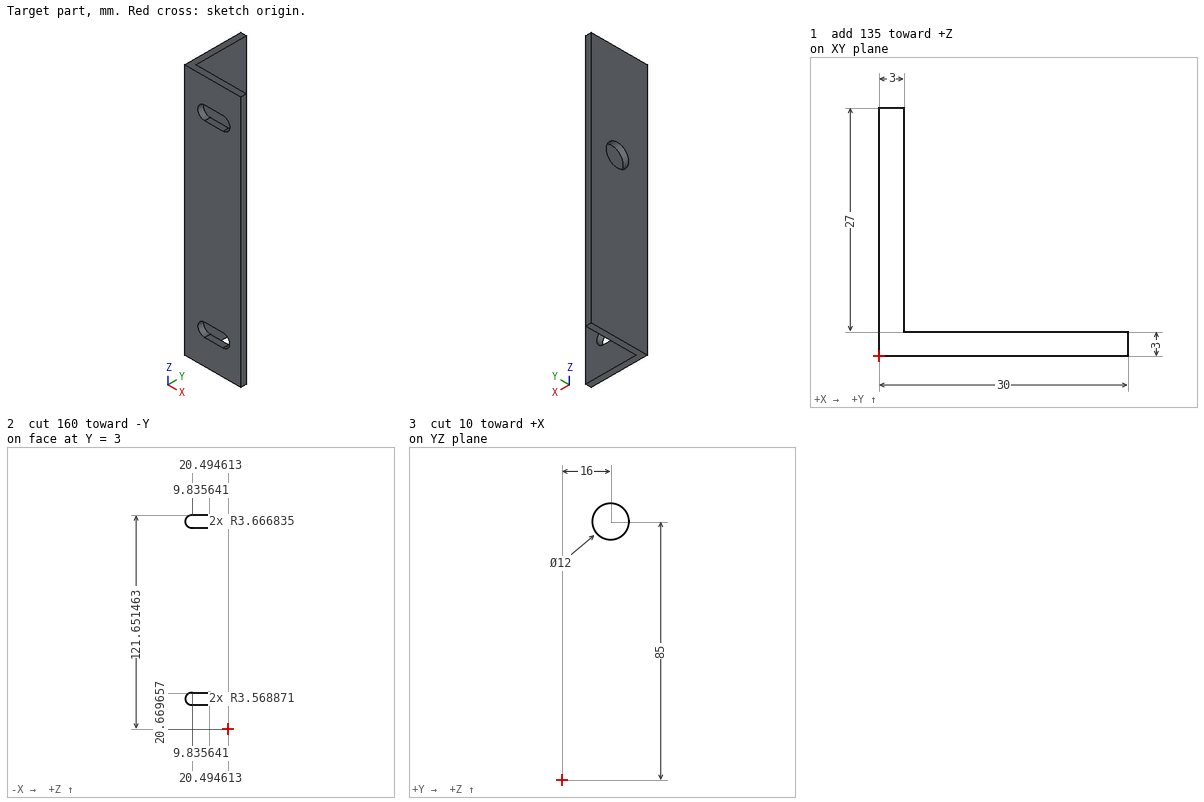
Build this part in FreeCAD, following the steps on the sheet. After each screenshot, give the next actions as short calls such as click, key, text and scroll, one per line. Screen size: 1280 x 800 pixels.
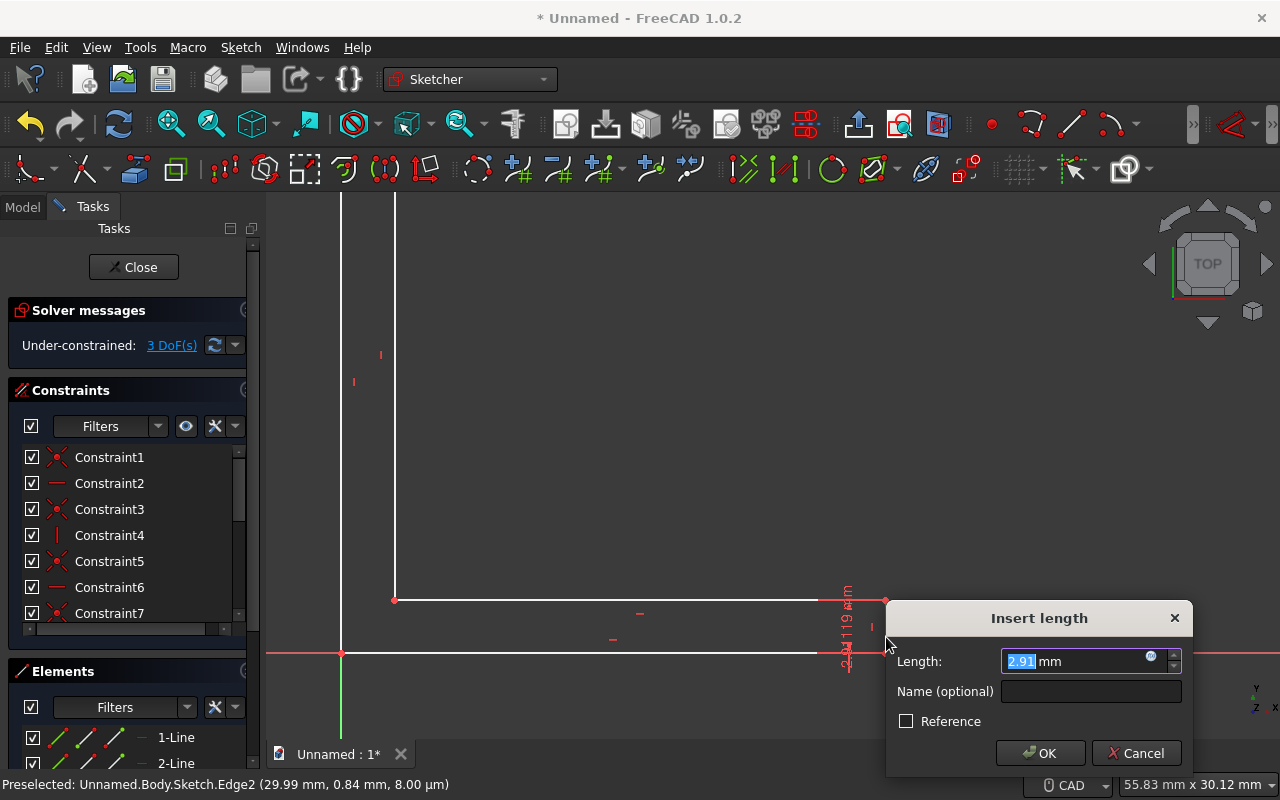
text(3)
key(Return)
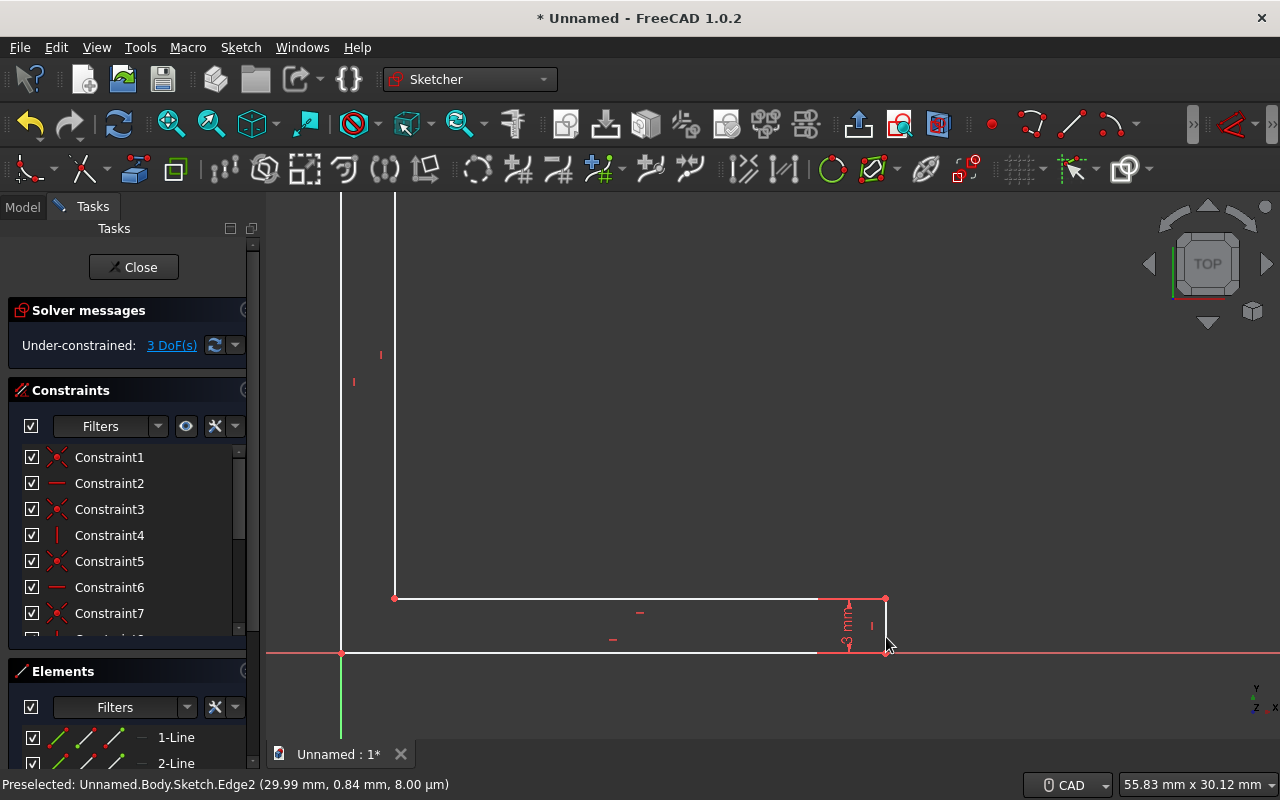
scroll(890, 638, down, 2)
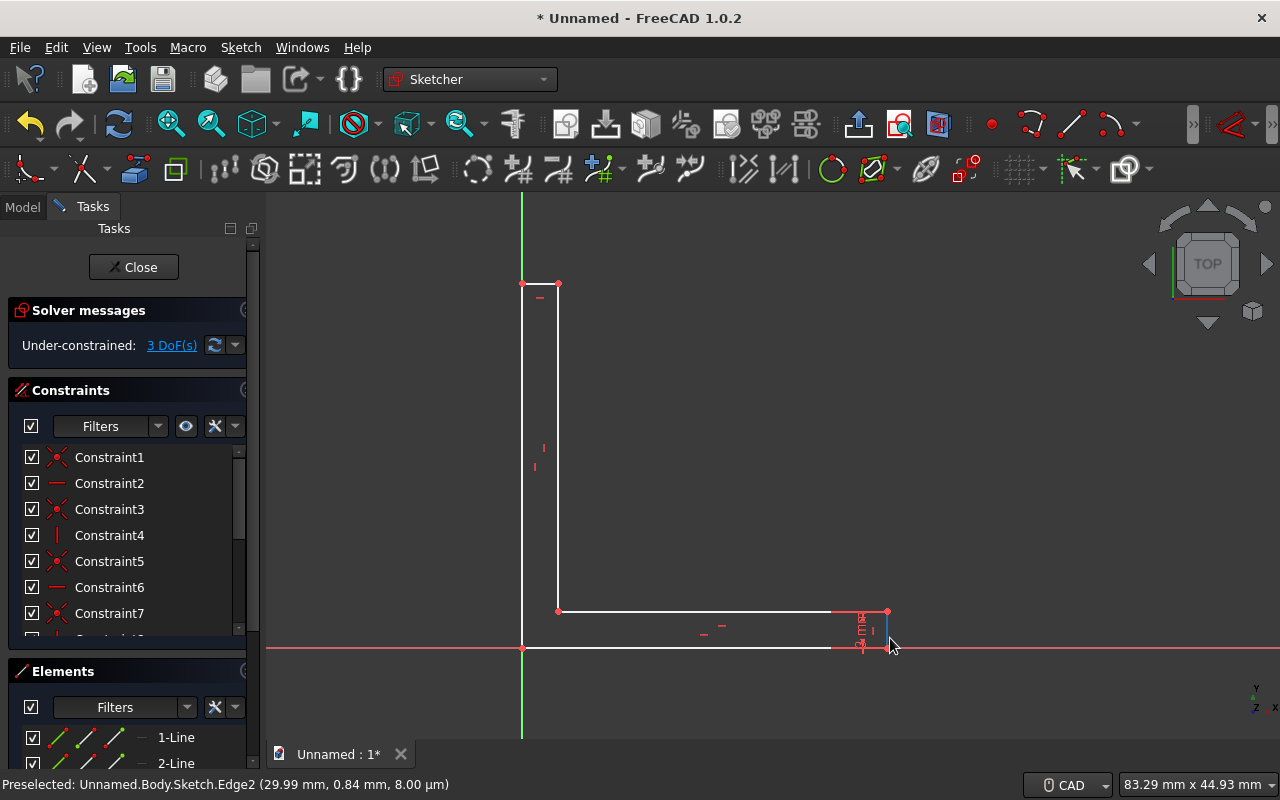
scroll(547, 284, up, 2)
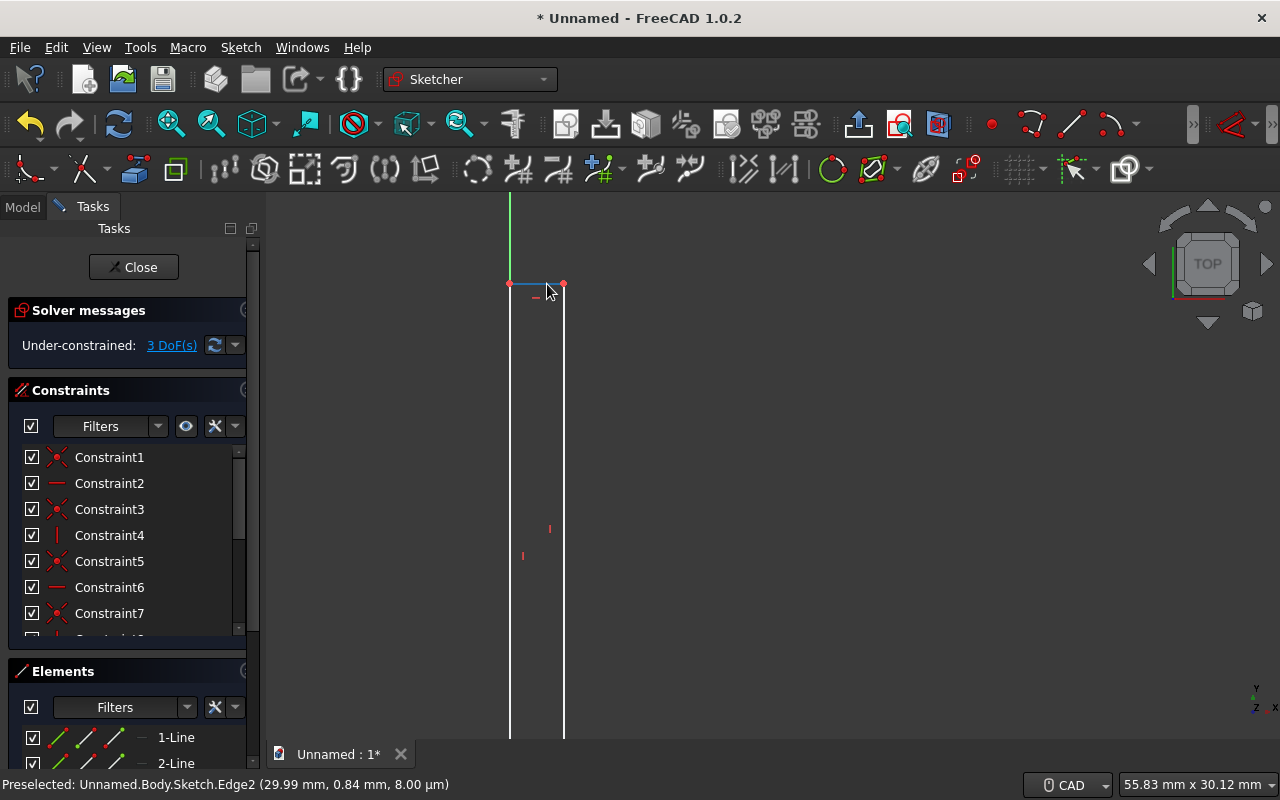
click(548, 284)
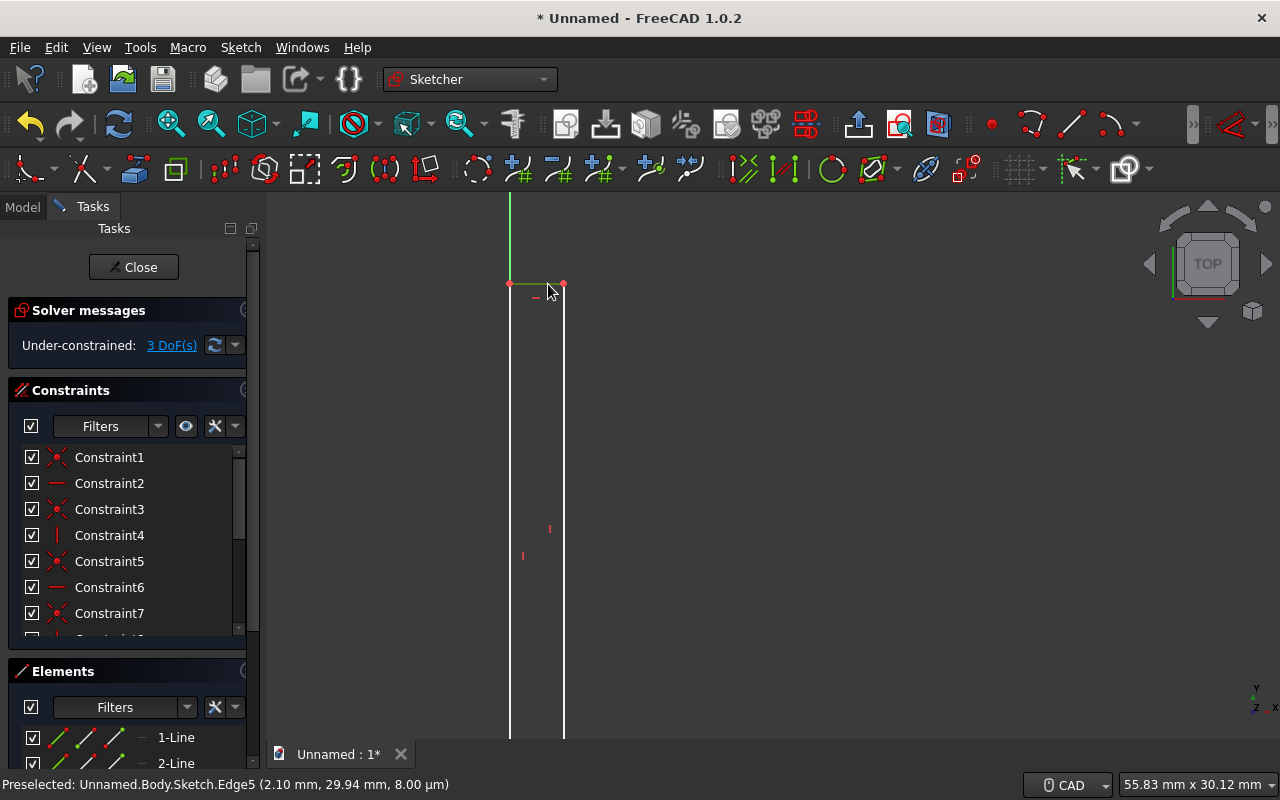
key(l)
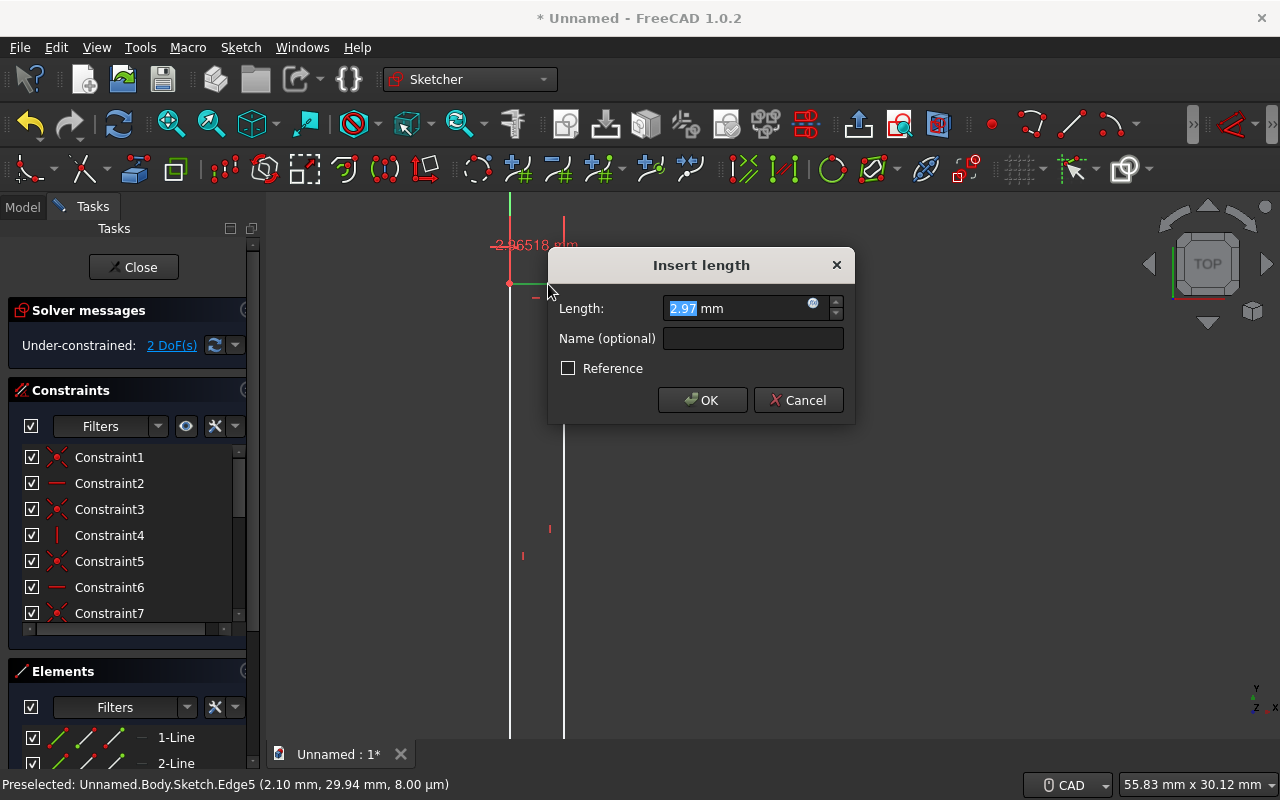
text(3)
key(Return)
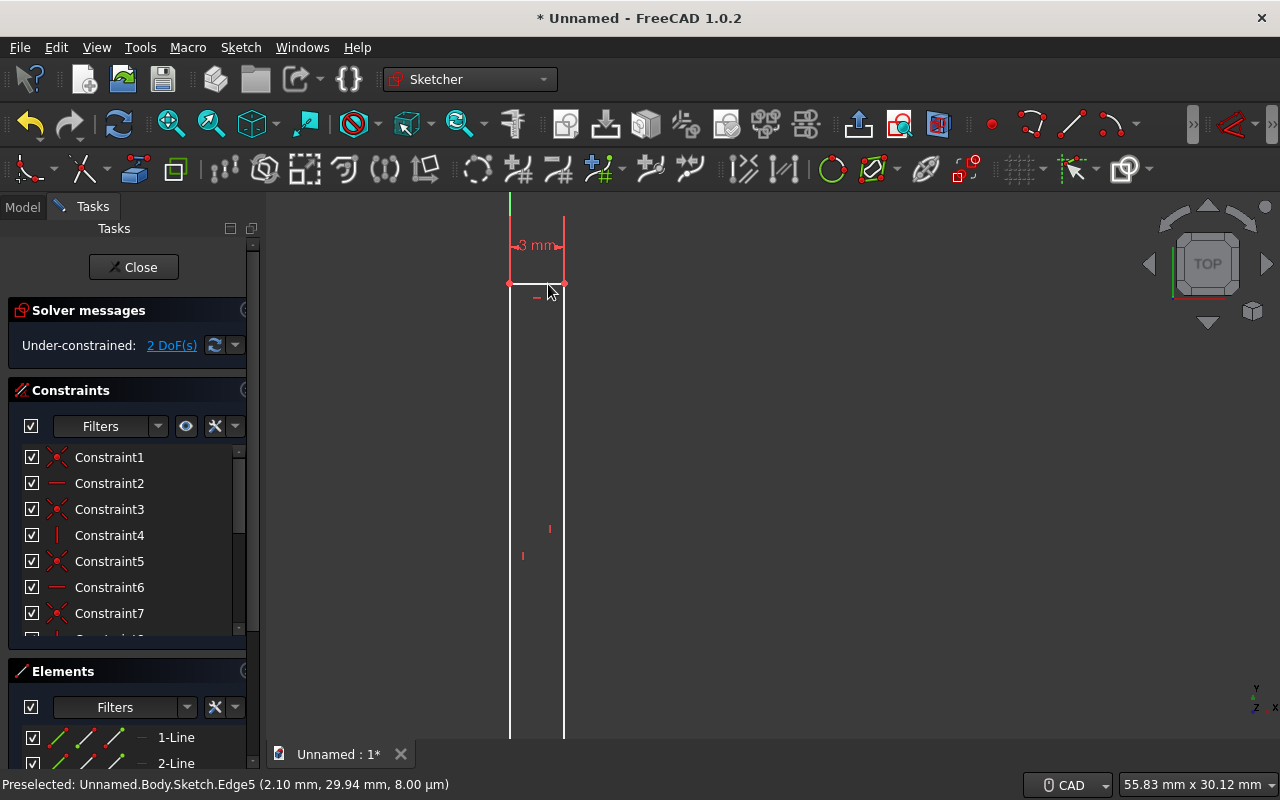
scroll(546, 283, down, 2)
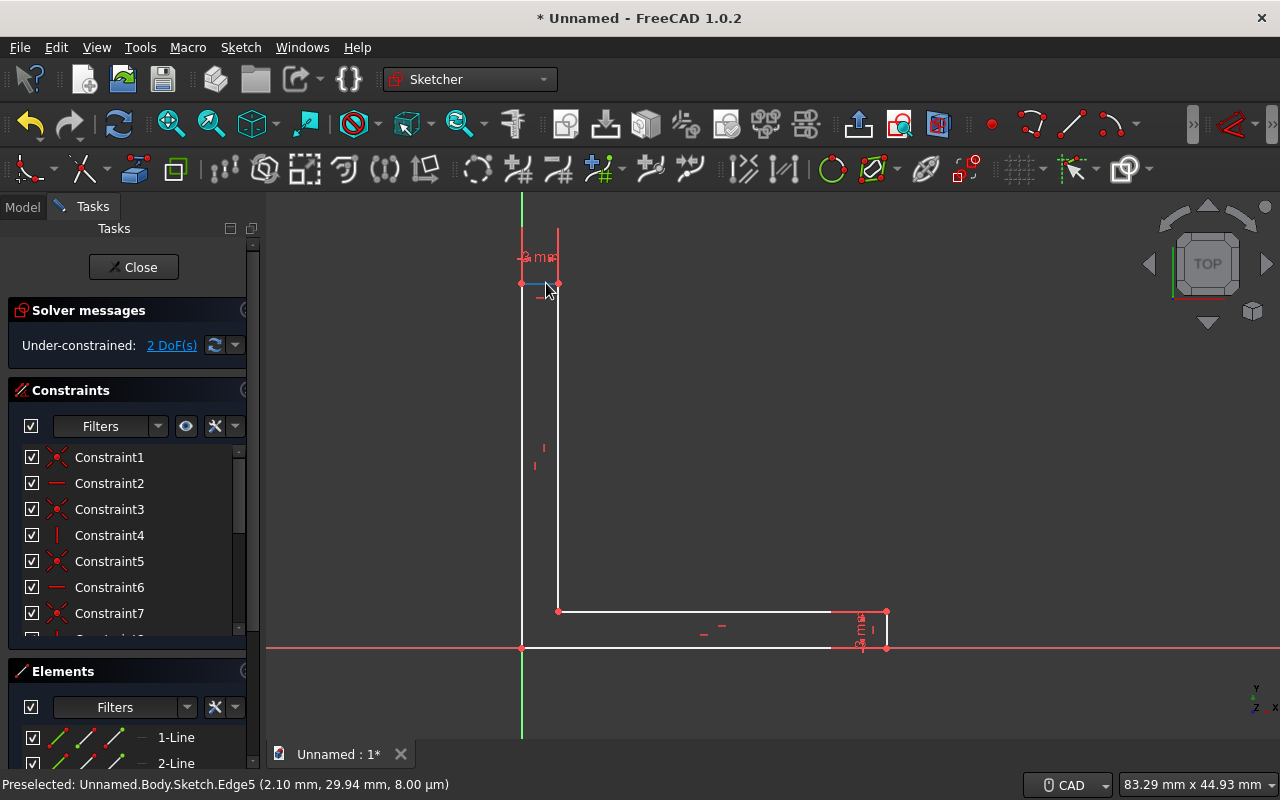
click(631, 648)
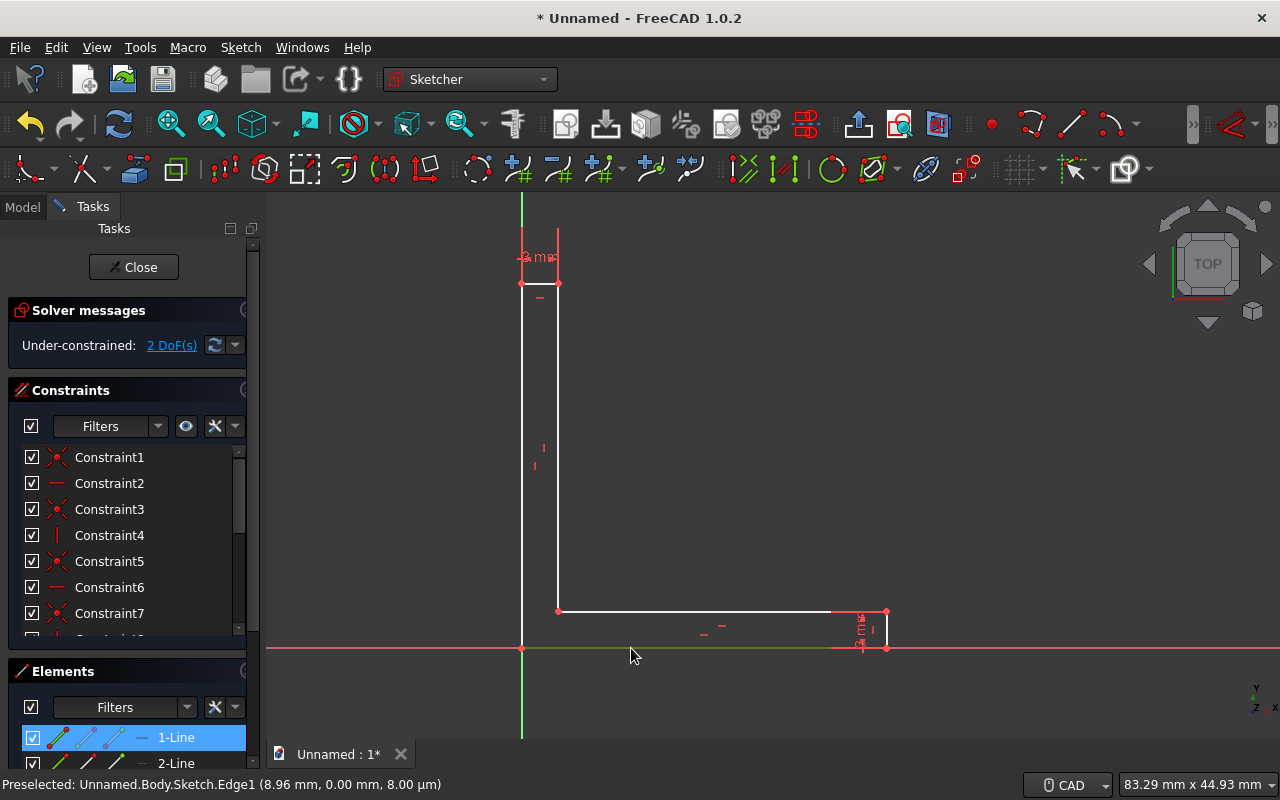
click(1258, 124)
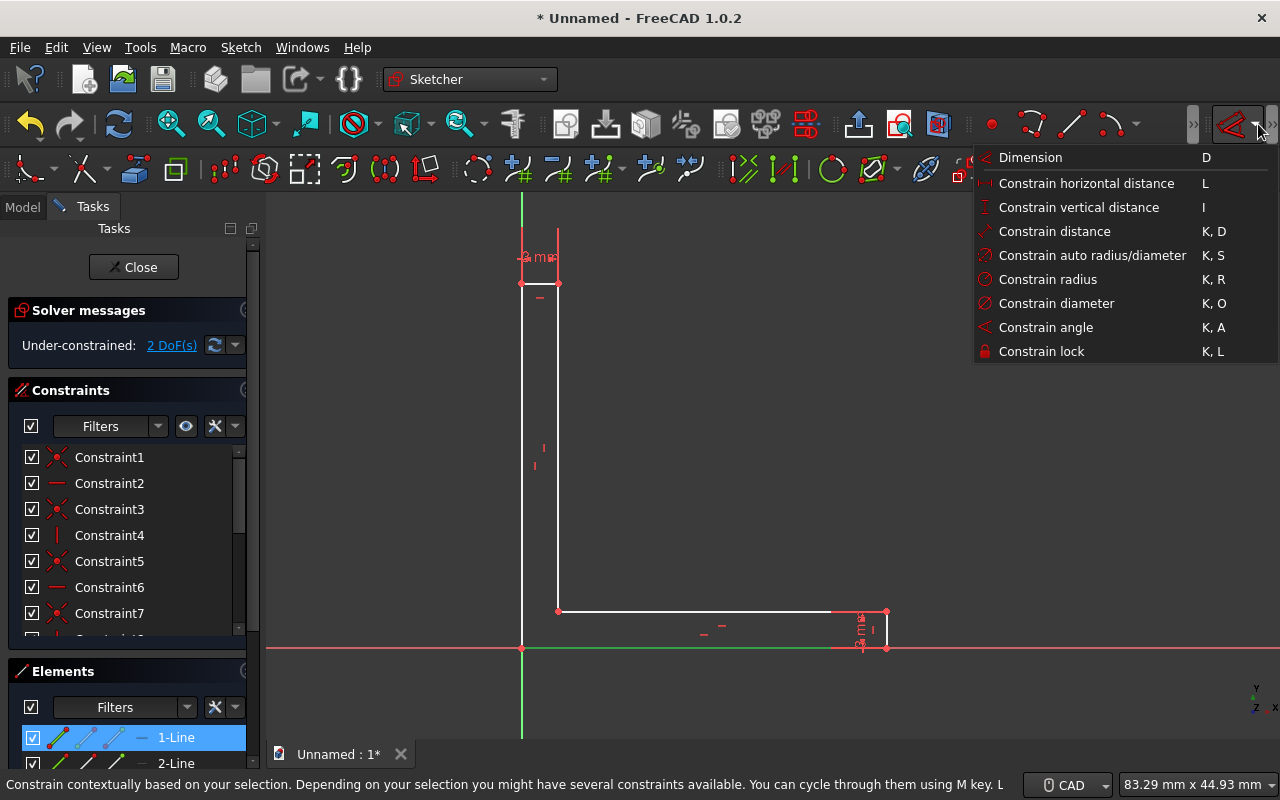
click(1126, 183)